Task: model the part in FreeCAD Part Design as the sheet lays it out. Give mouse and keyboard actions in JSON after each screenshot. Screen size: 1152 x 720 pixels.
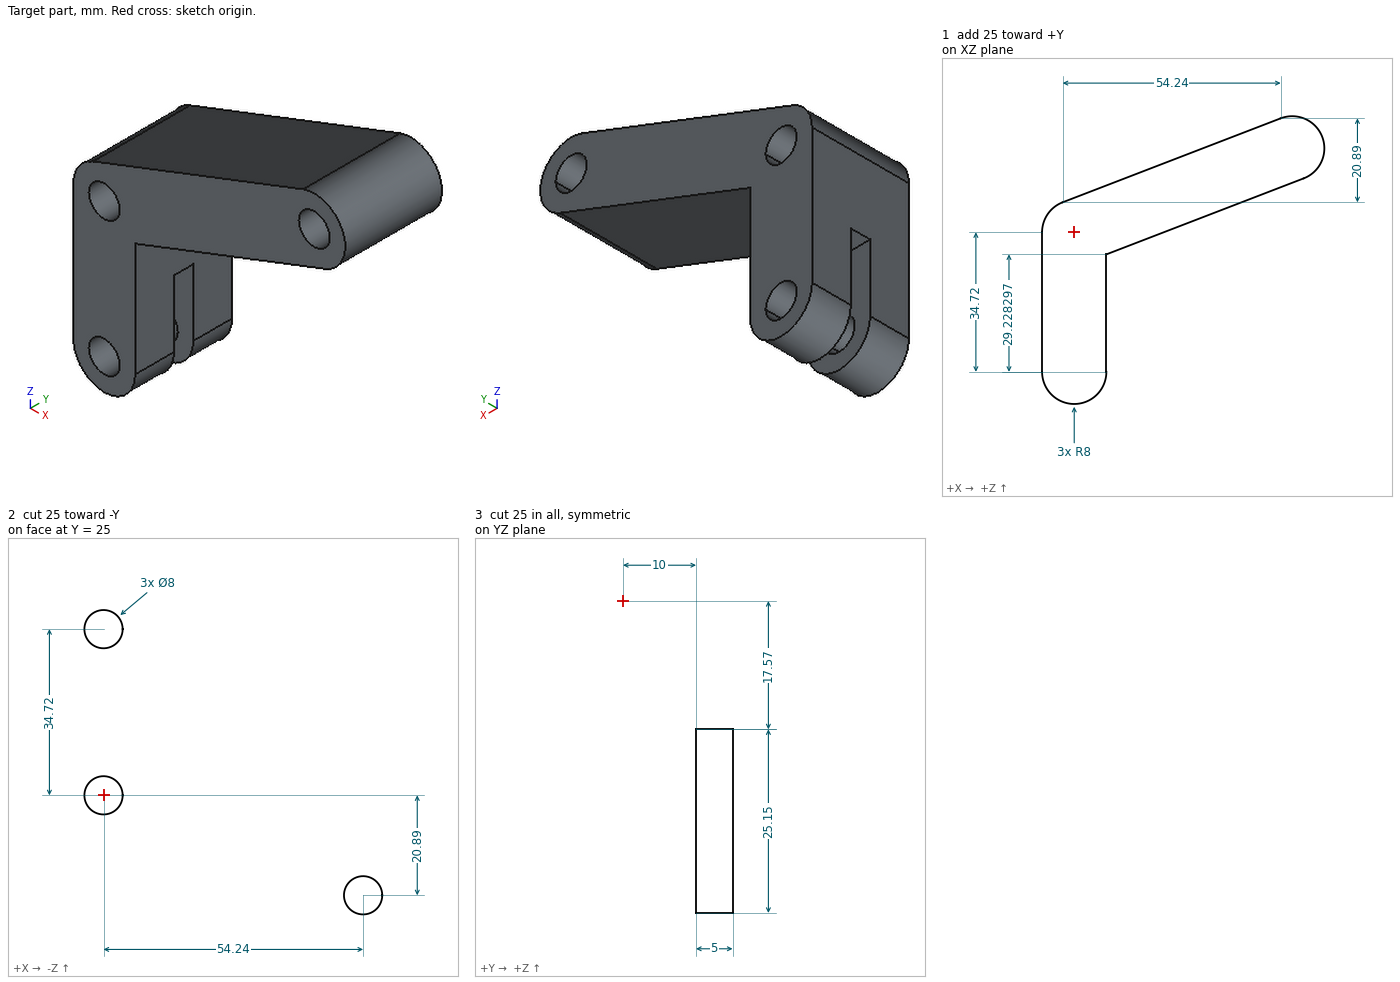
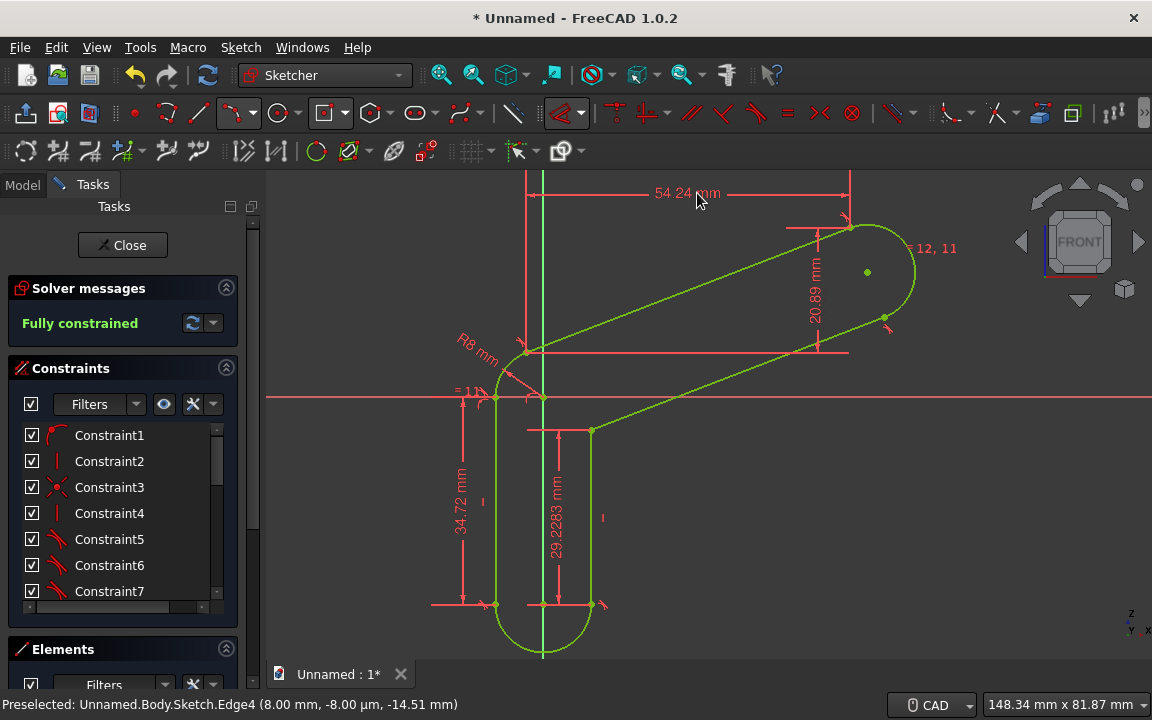
{"action": "left_click", "coordinate": [123, 245]}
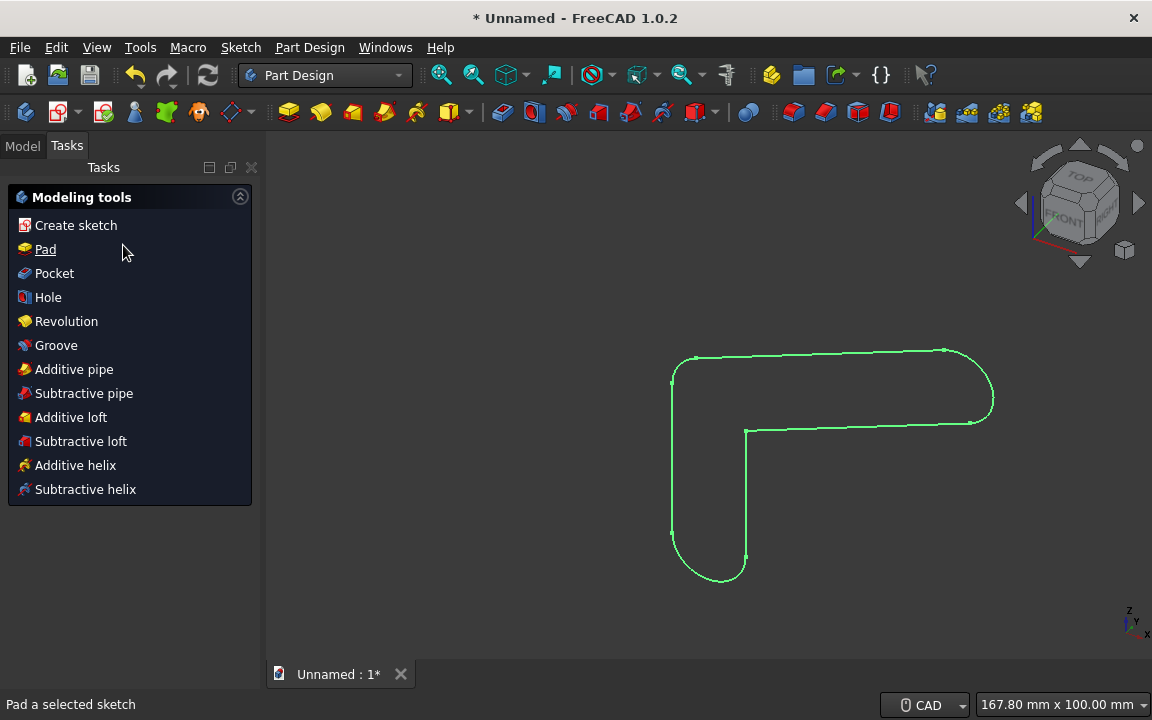
{"action": "left_click", "coordinate": [290, 112]}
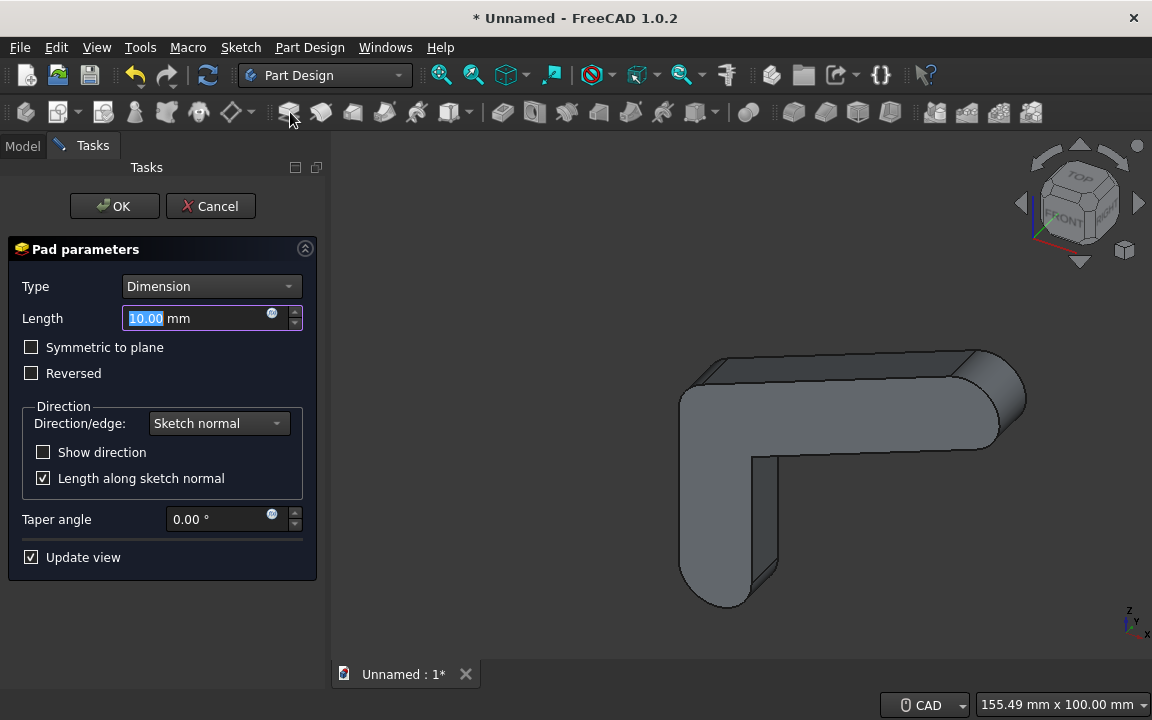
{"action": "type", "text": "25"}
{"action": "key", "text": "Tab"}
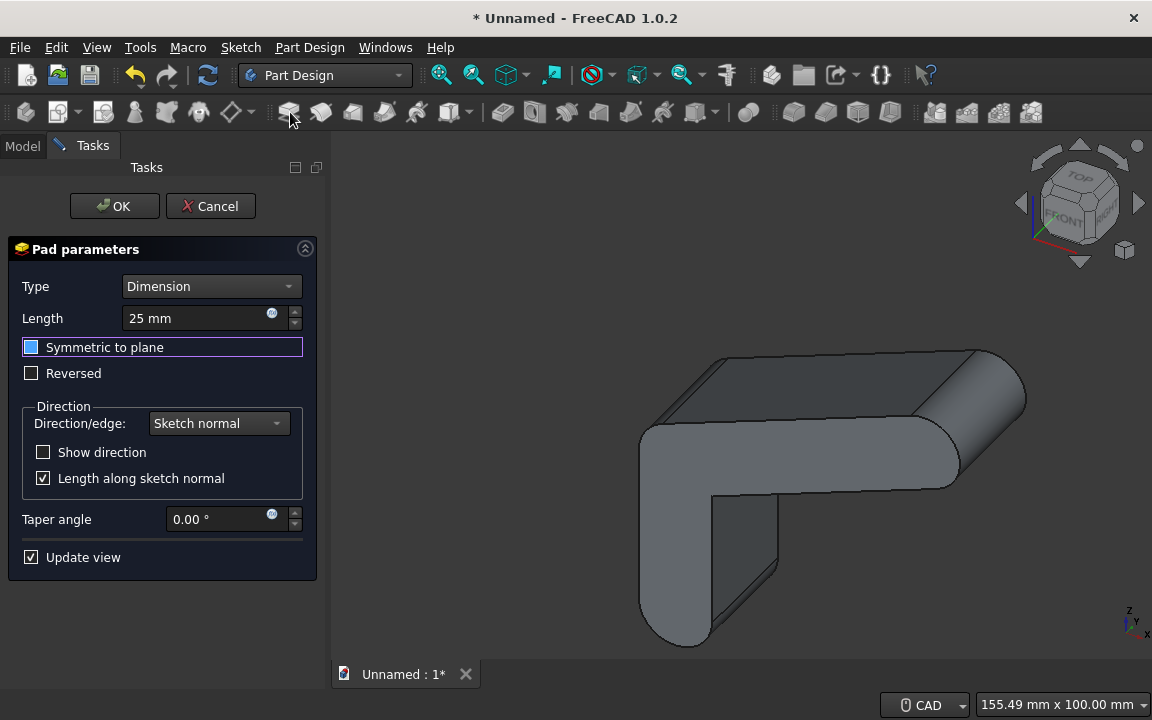
{"action": "left_click", "coordinate": [30, 373]}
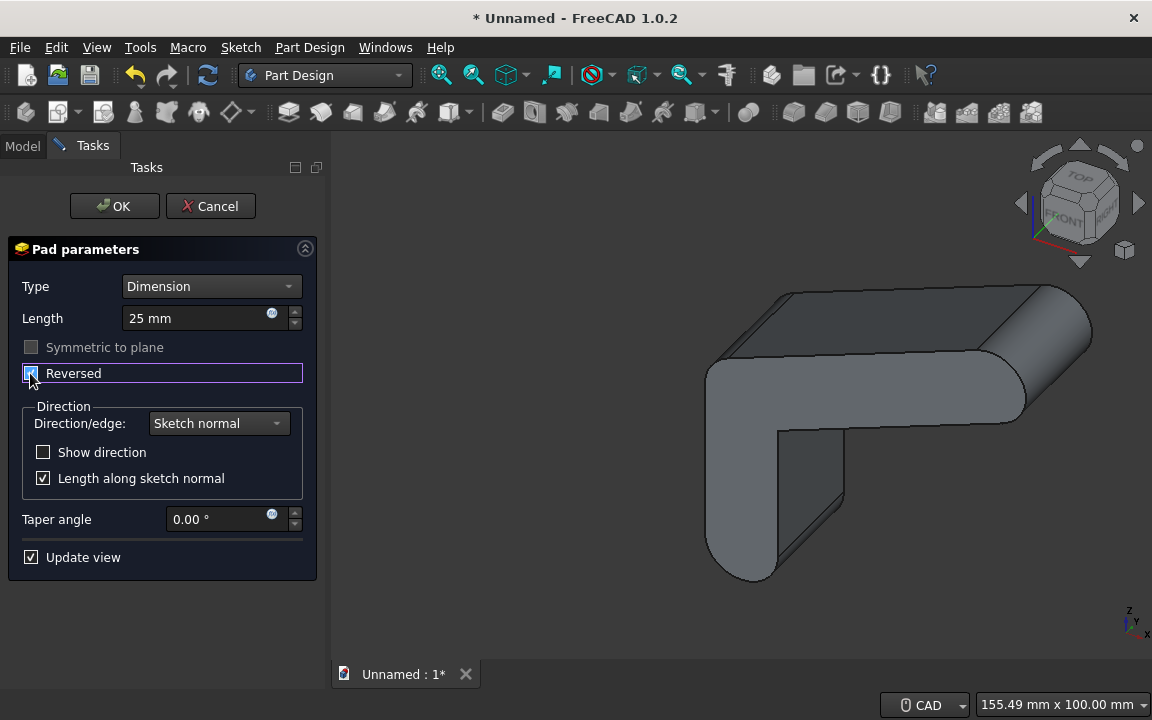
{"action": "left_click", "coordinate": [115, 206]}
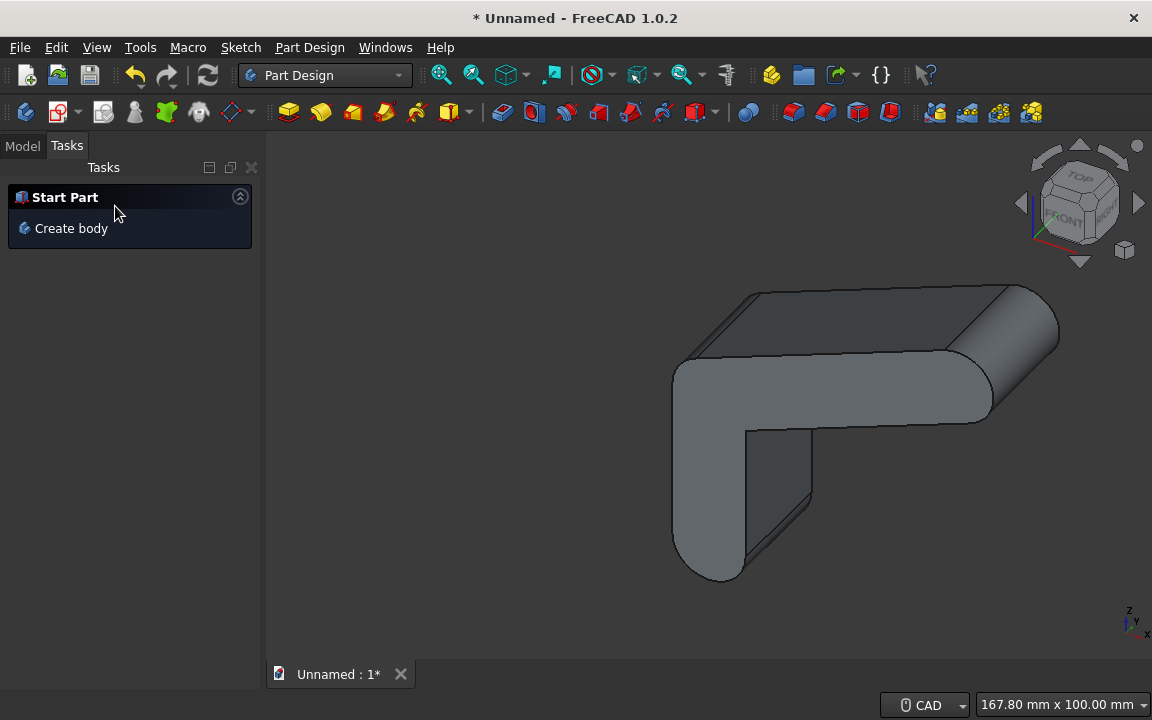
{"action": "left_click", "coordinate": [442, 76]}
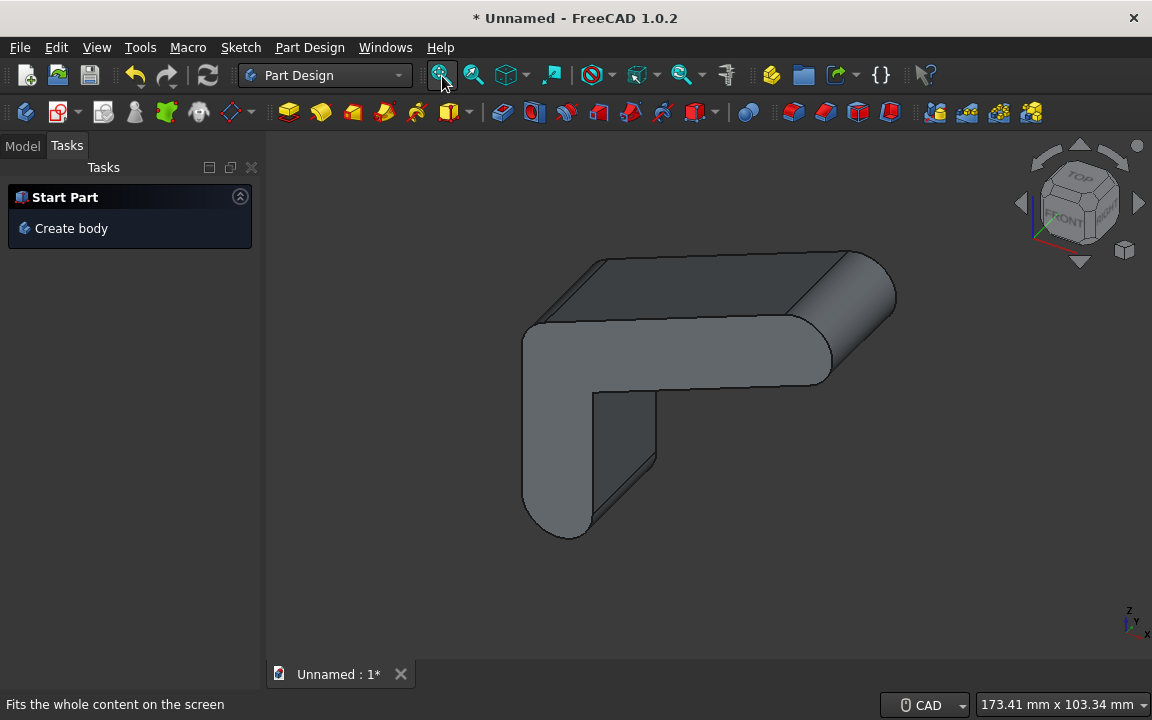
{"action": "key", "text": "4"}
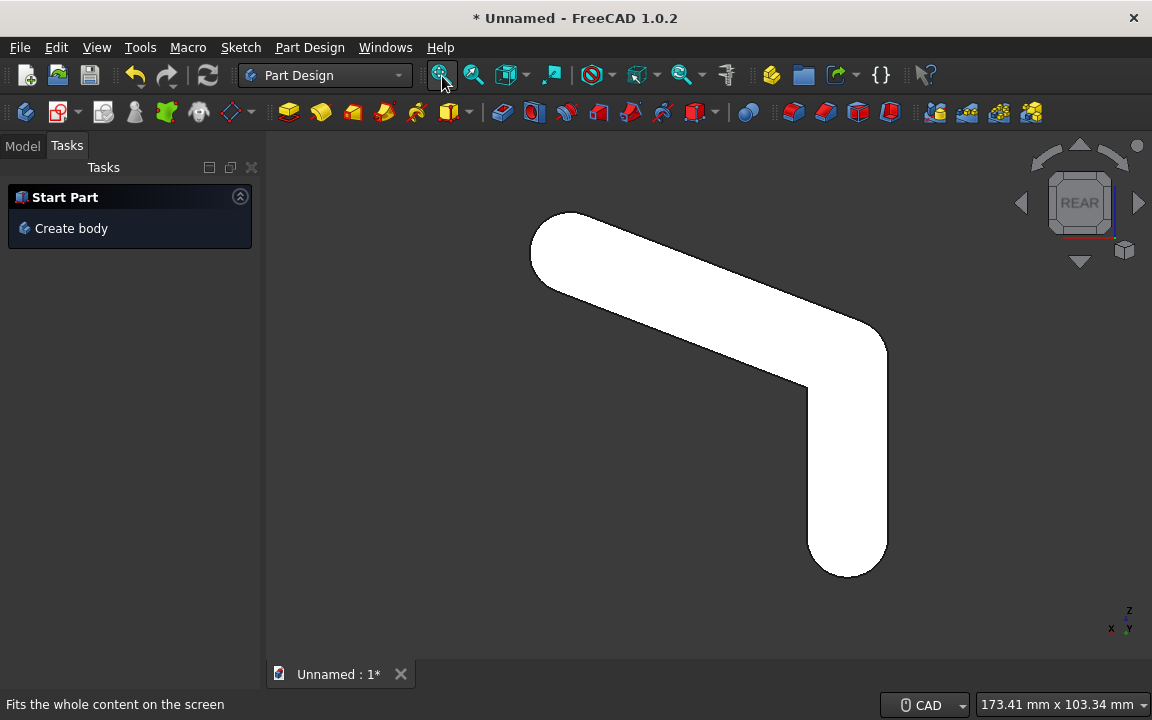
{"action": "left_click", "coordinate": [811, 342]}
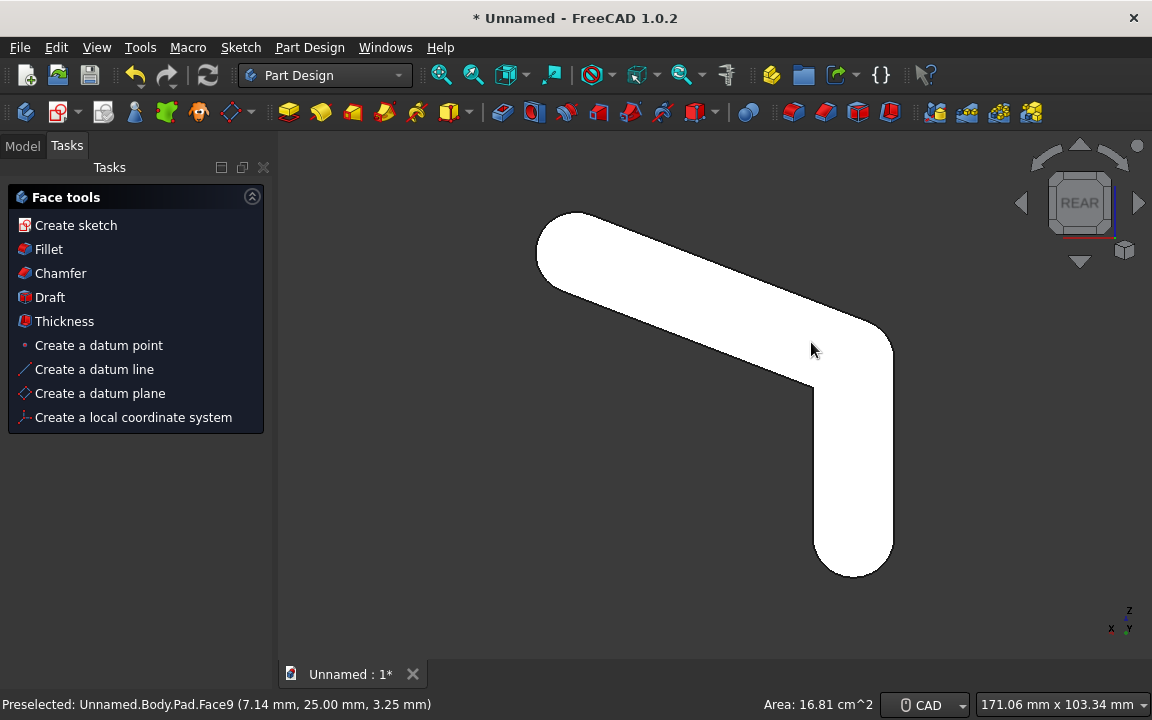
{"action": "left_click", "coordinate": [58, 112]}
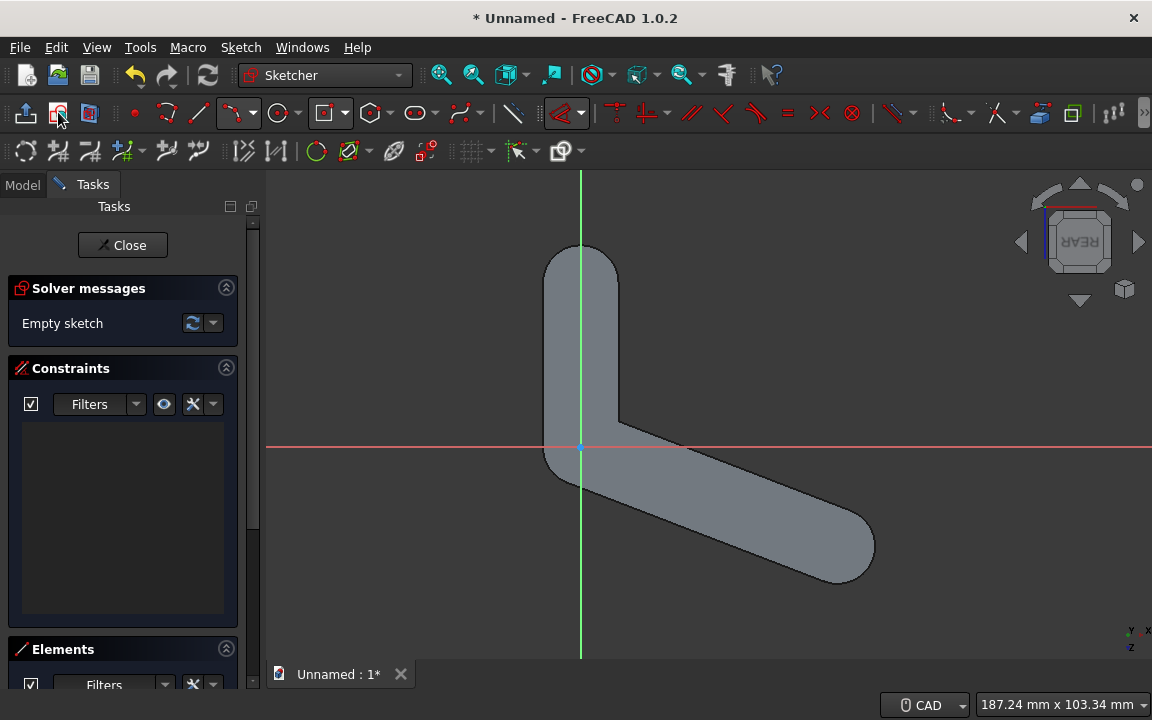
{"action": "left_click", "coordinate": [278, 114]}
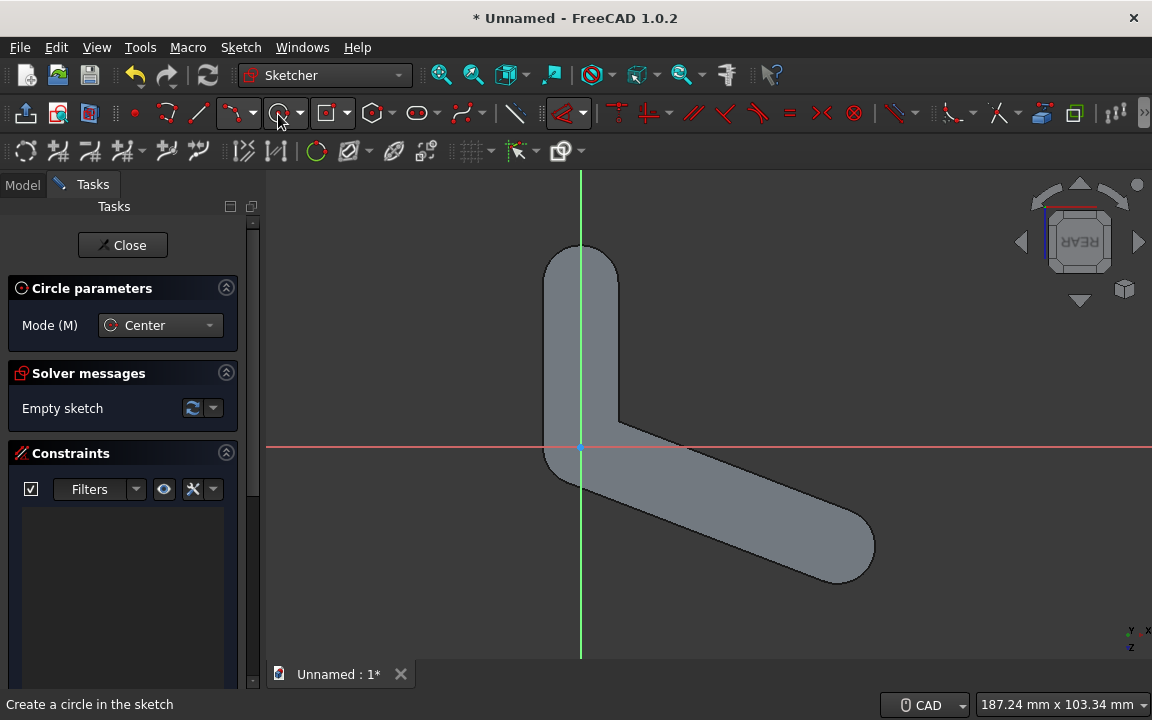
{"action": "left_click", "coordinate": [581, 283]}
{"action": "left_click", "coordinate": [599, 277]}